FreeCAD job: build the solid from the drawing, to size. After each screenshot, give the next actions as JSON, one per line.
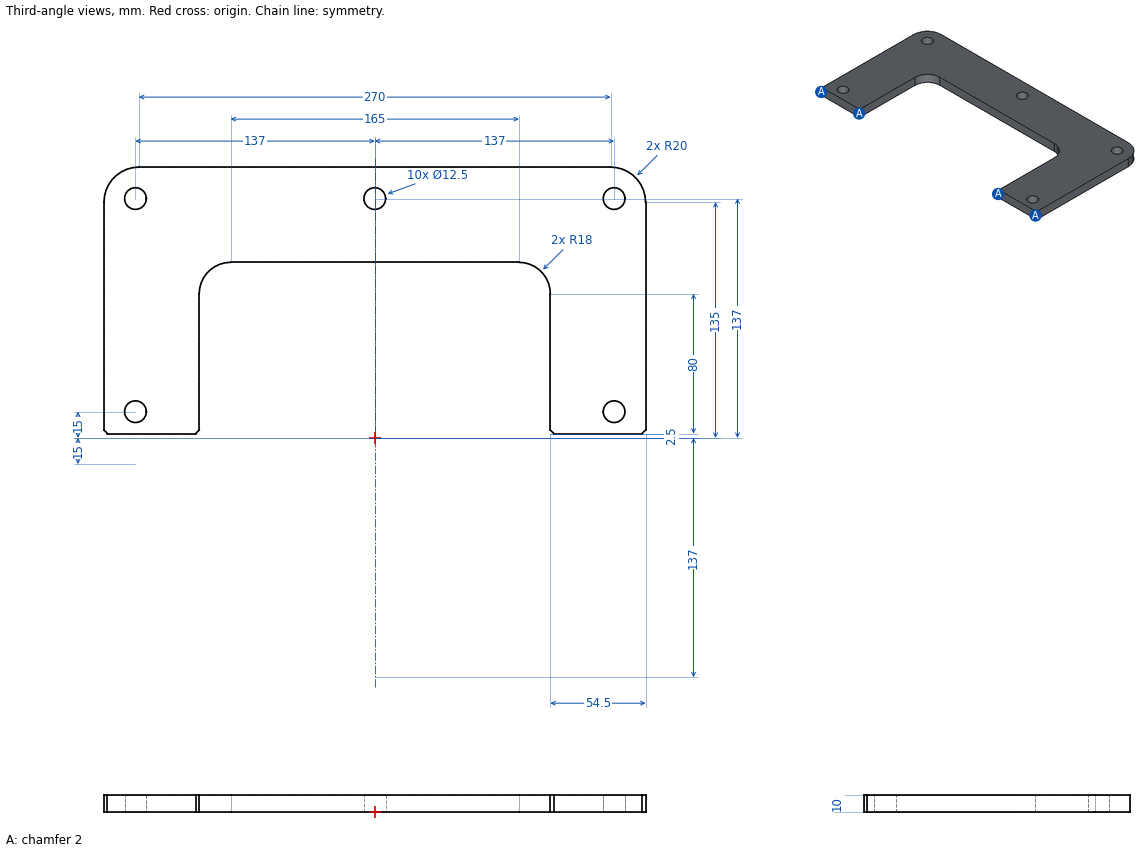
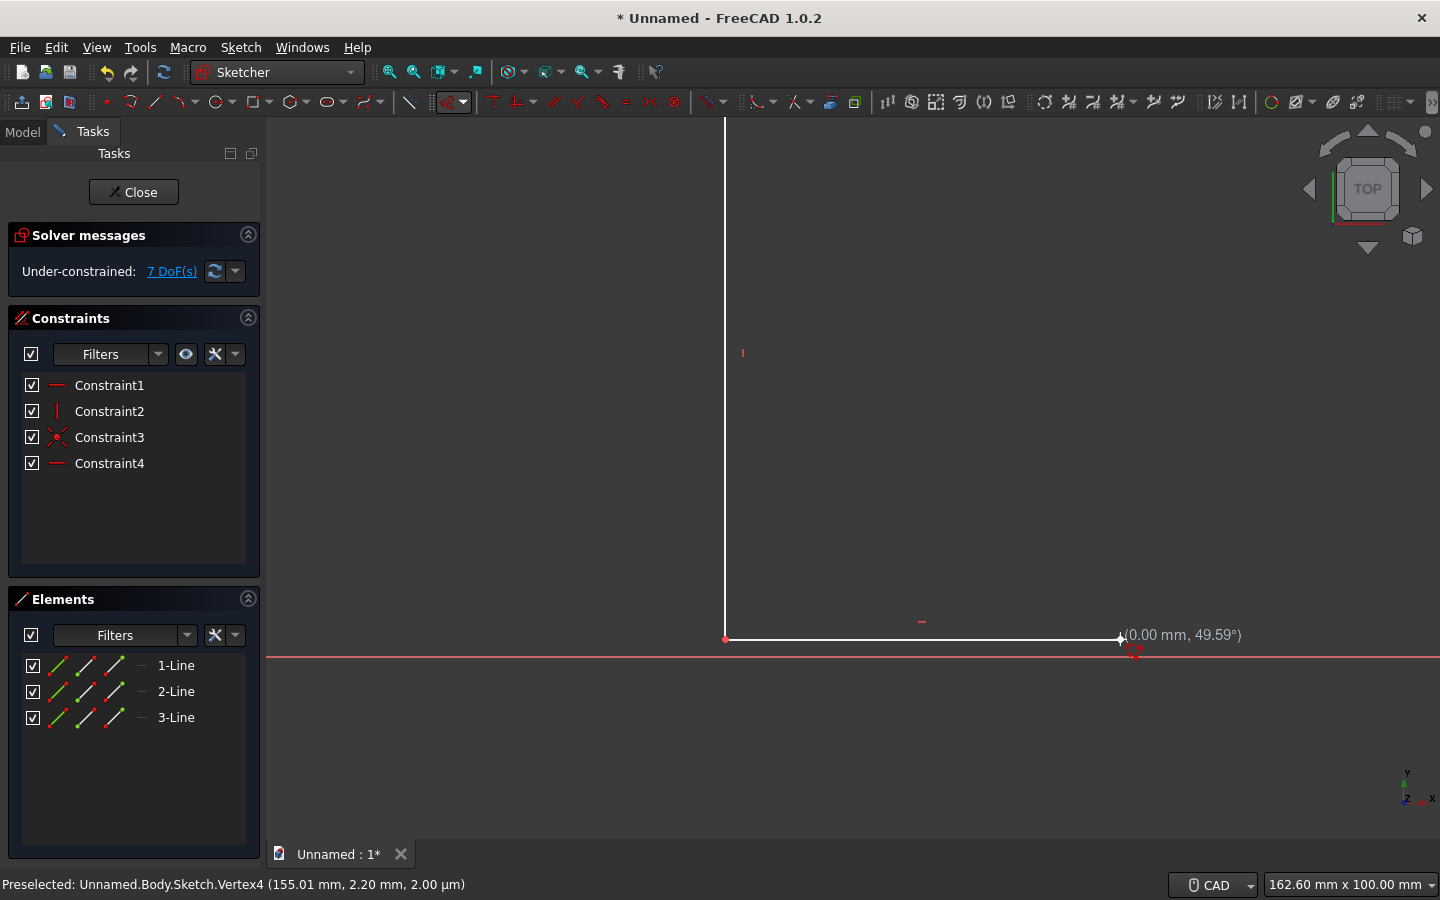
{"action": "scroll", "coordinate": [1122, 642], "scroll_direction": "down", "scroll_amount": 6}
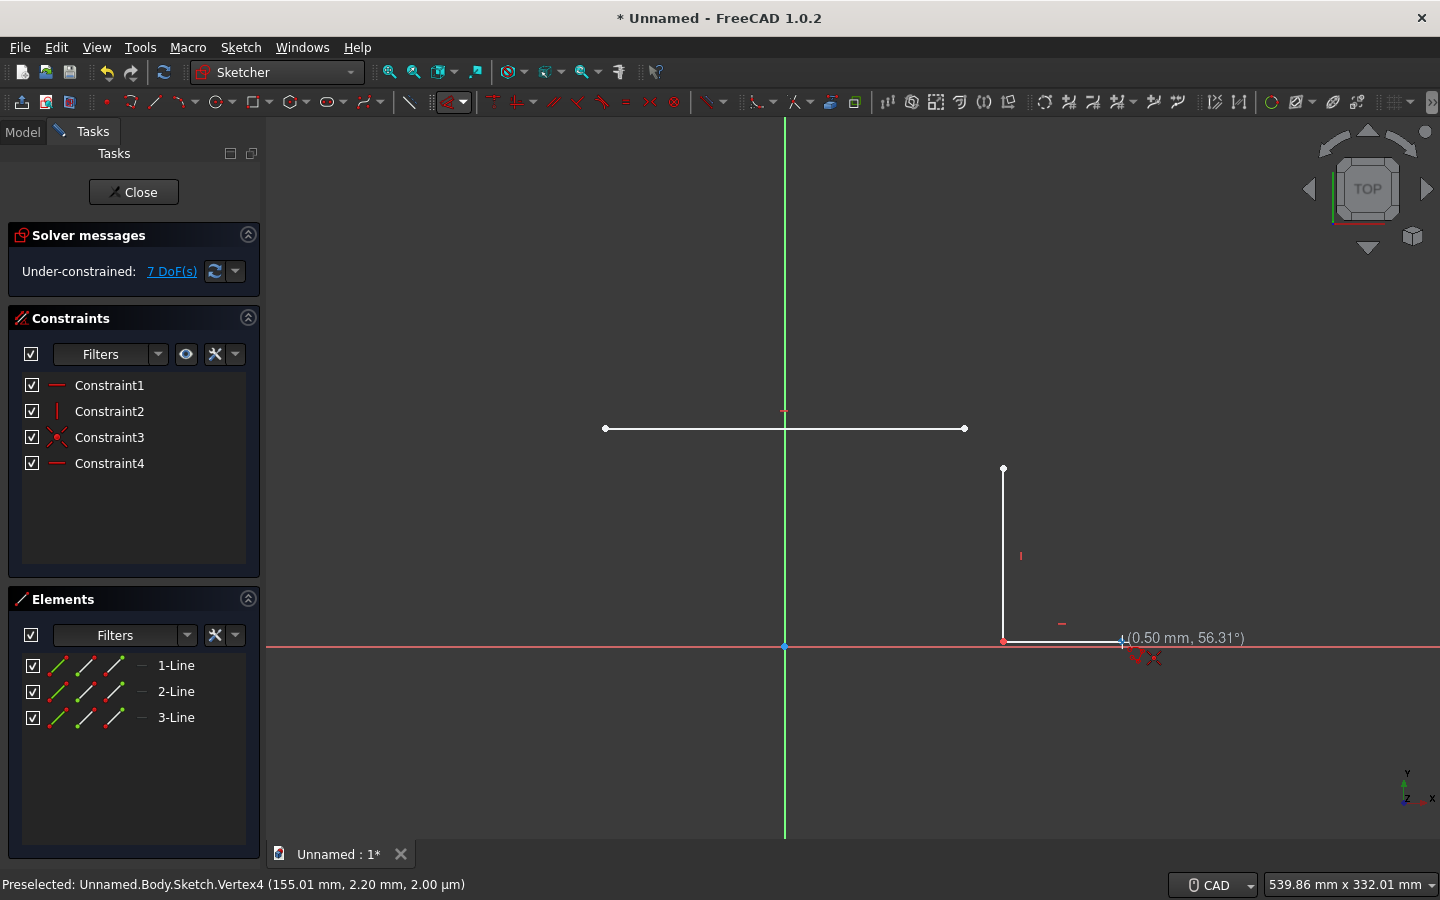
{"action": "left_click", "coordinate": [1122, 353]}
{"action": "right_click", "coordinate": [1122, 353]}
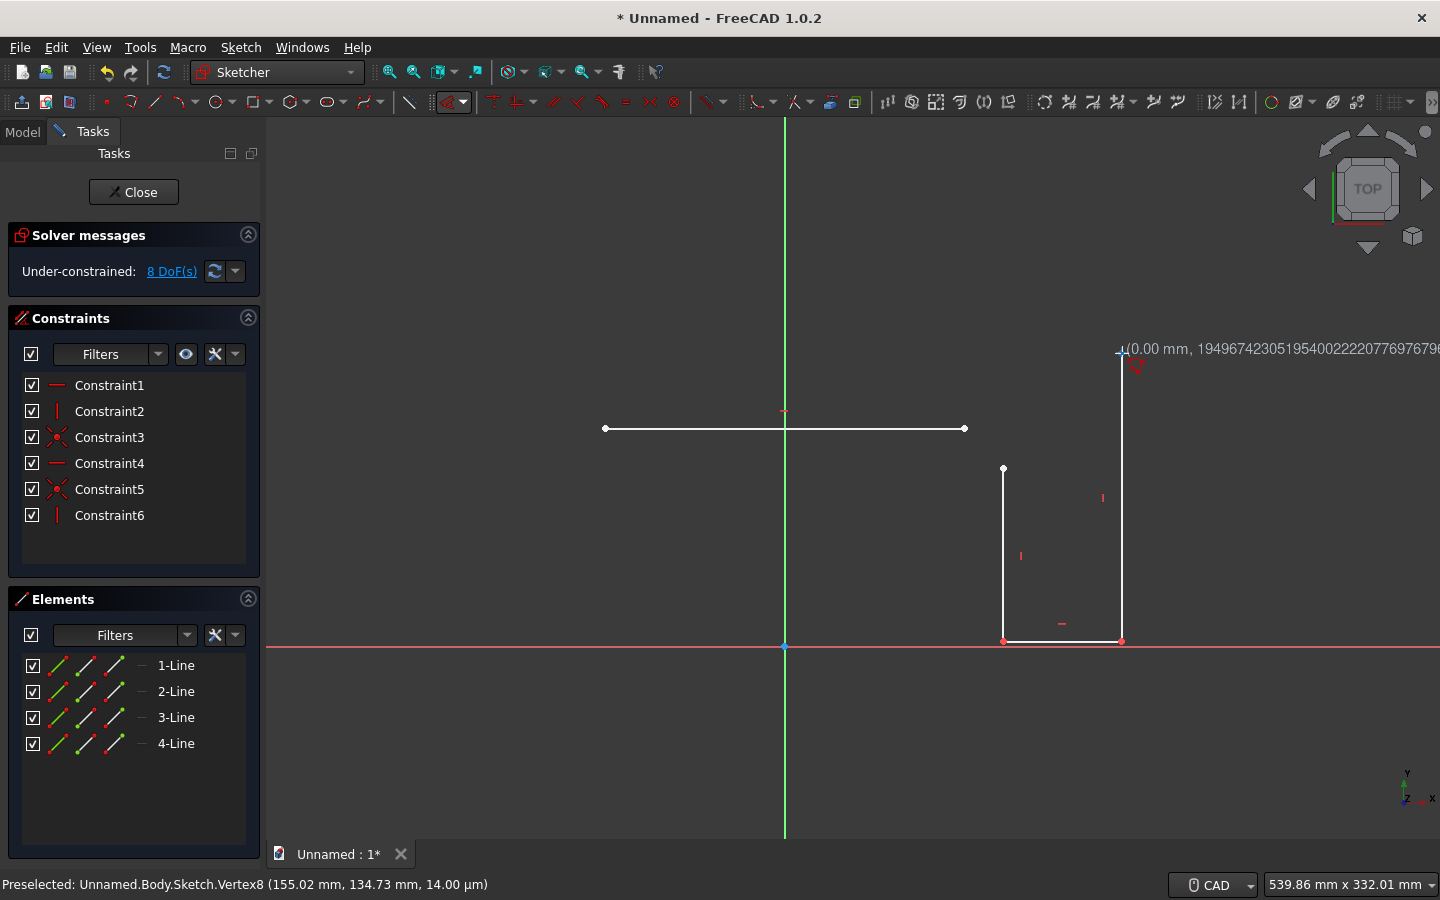
{"action": "key", "text": "g l"}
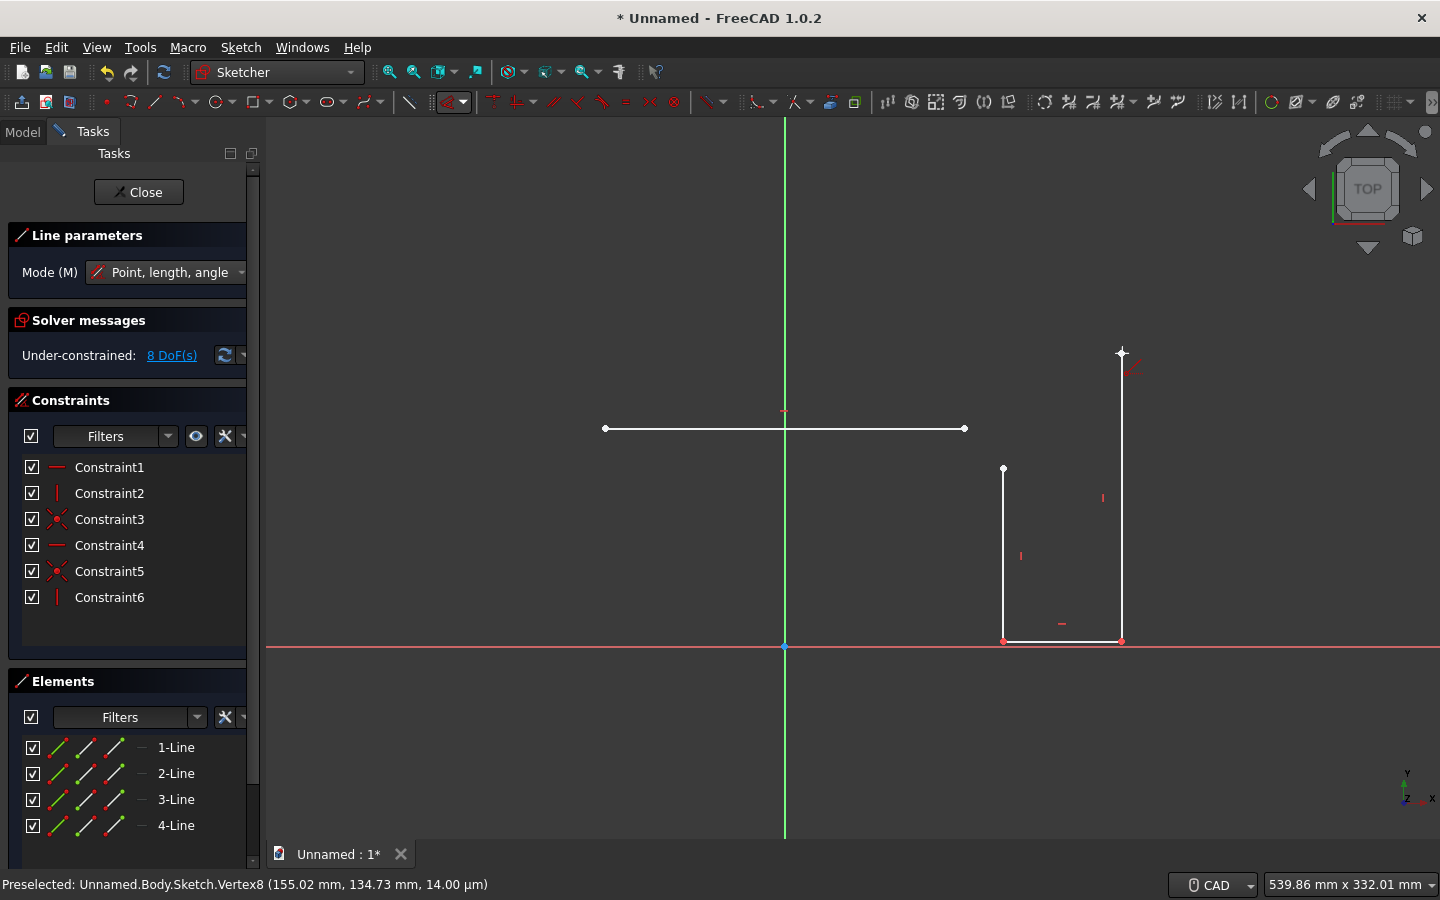
{"action": "left_click", "coordinate": [1078, 310]}
{"action": "left_click", "coordinate": [491, 310]}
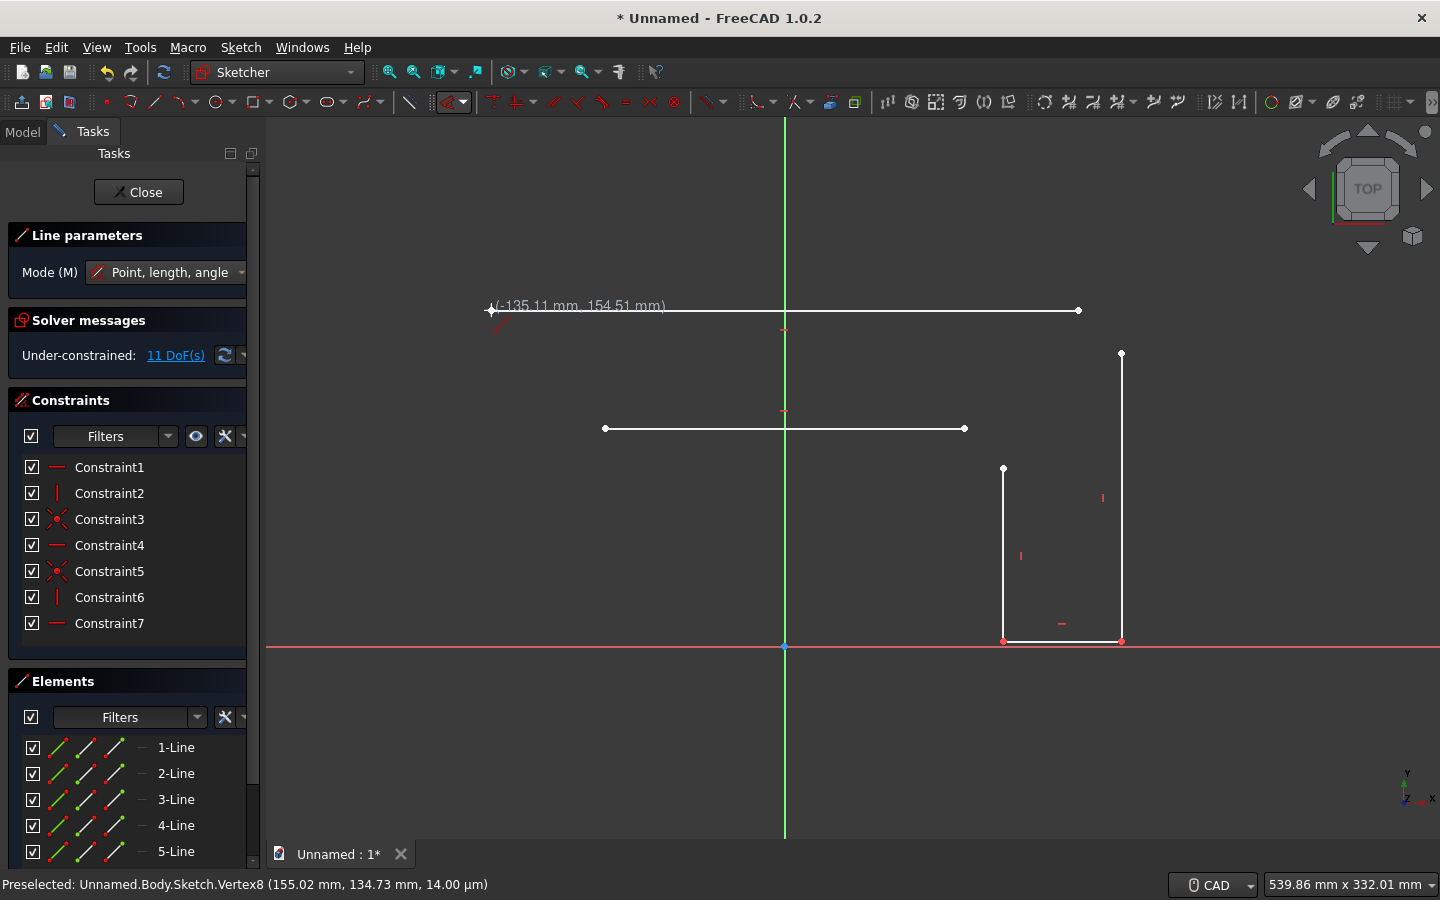
{"action": "key", "text": "g m"}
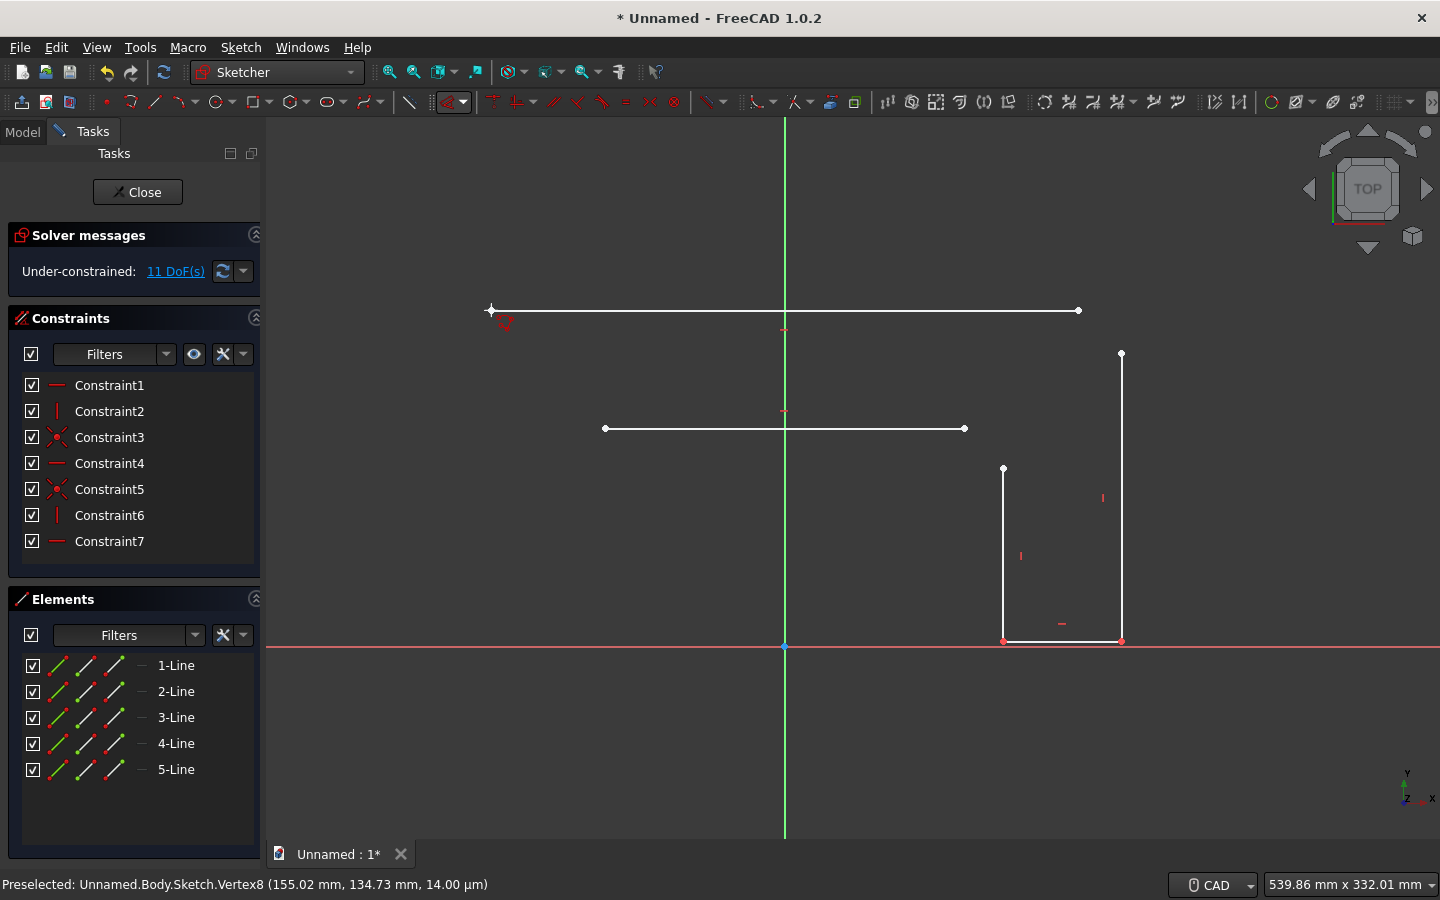
{"action": "left_click", "coordinate": [448, 353]}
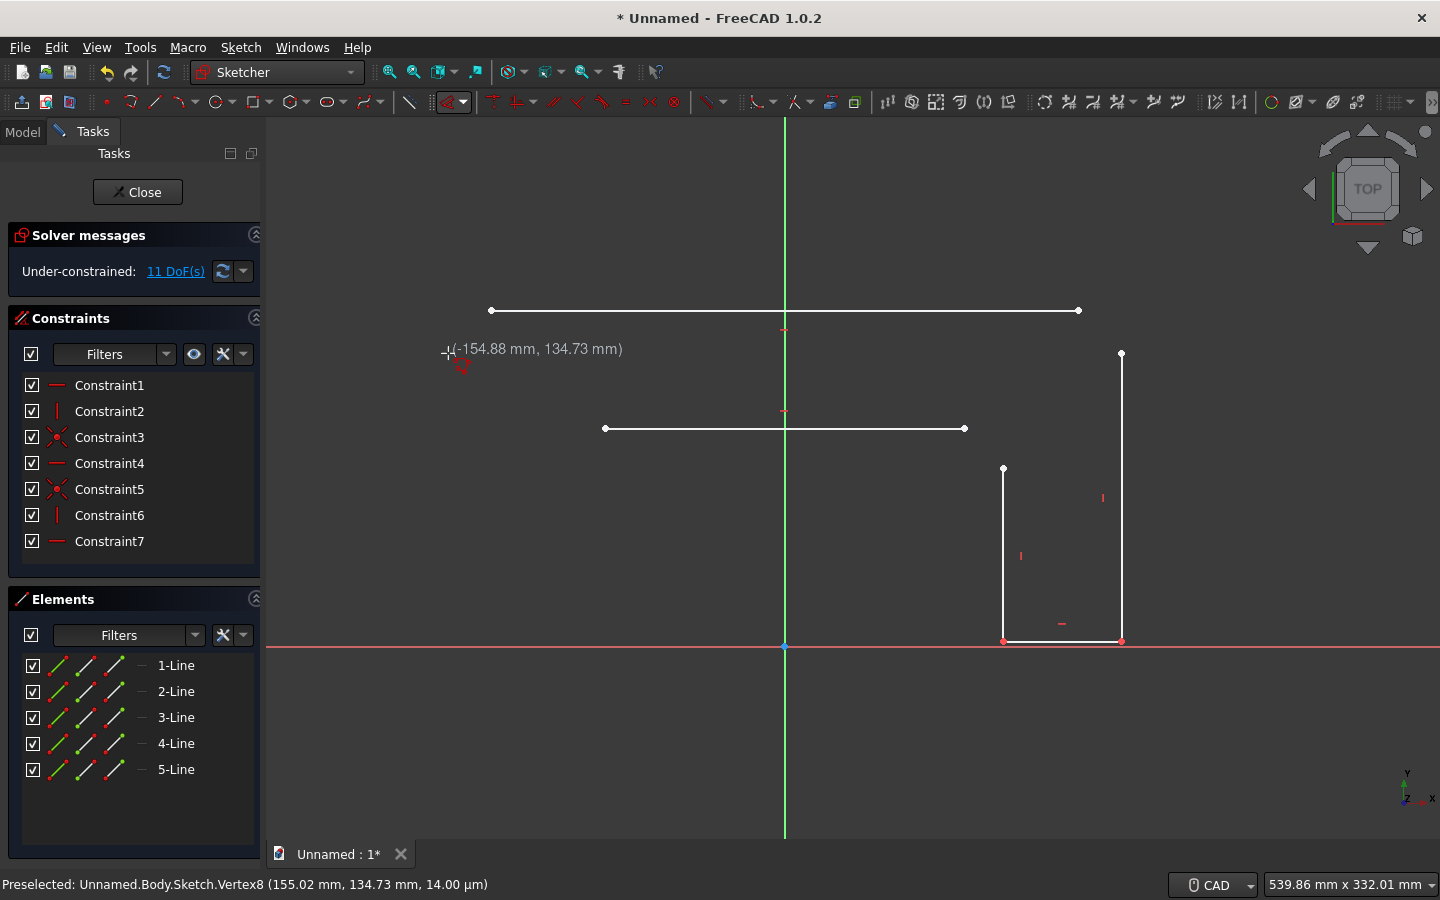
{"action": "scroll", "coordinate": [448, 642], "scroll_direction": "up", "scroll_amount": 6}